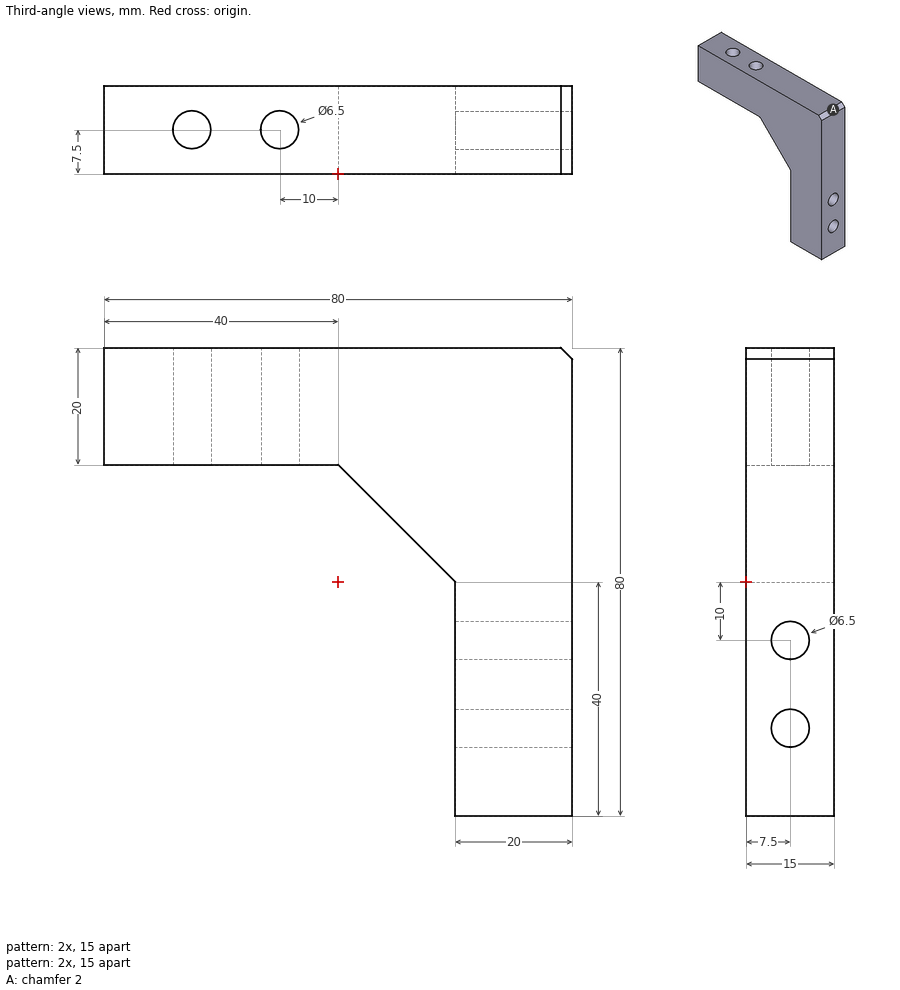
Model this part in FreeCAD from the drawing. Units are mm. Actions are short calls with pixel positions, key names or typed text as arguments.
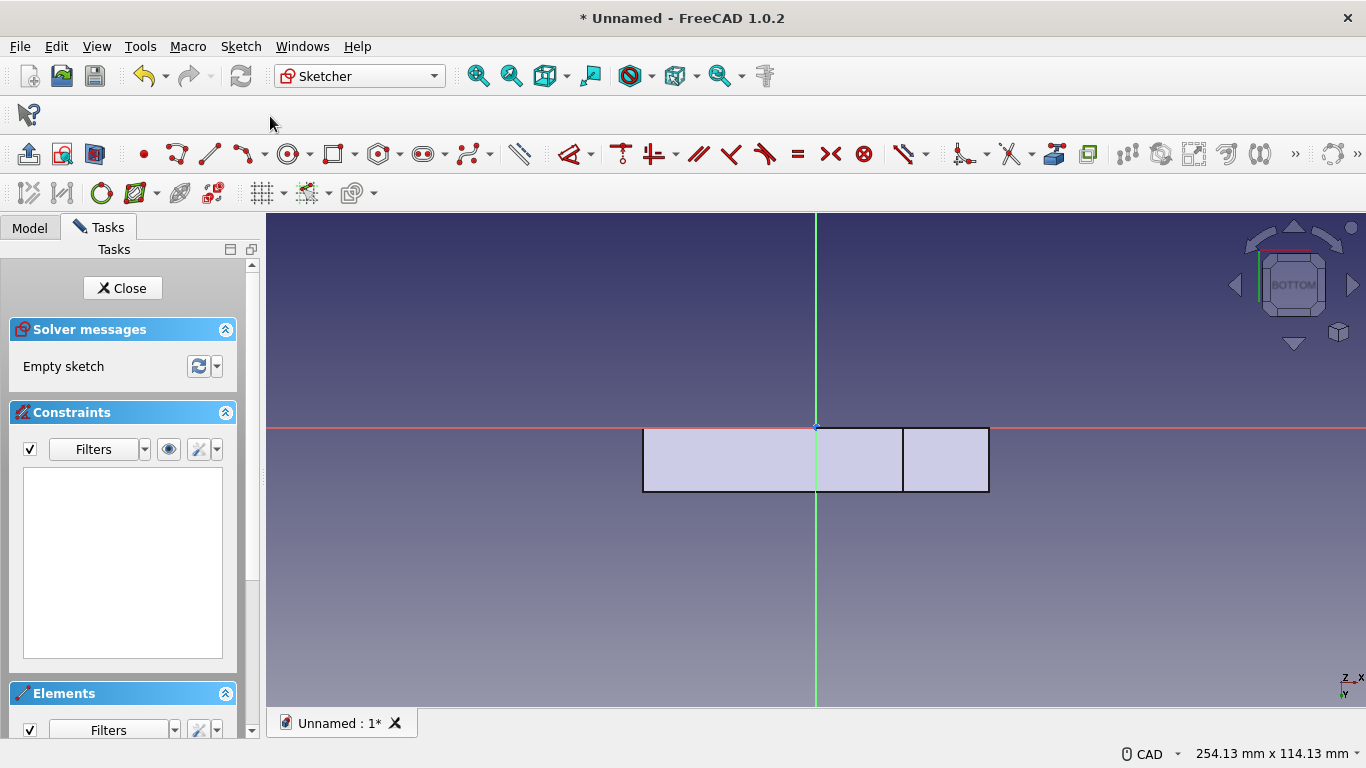
key(q)
key(s)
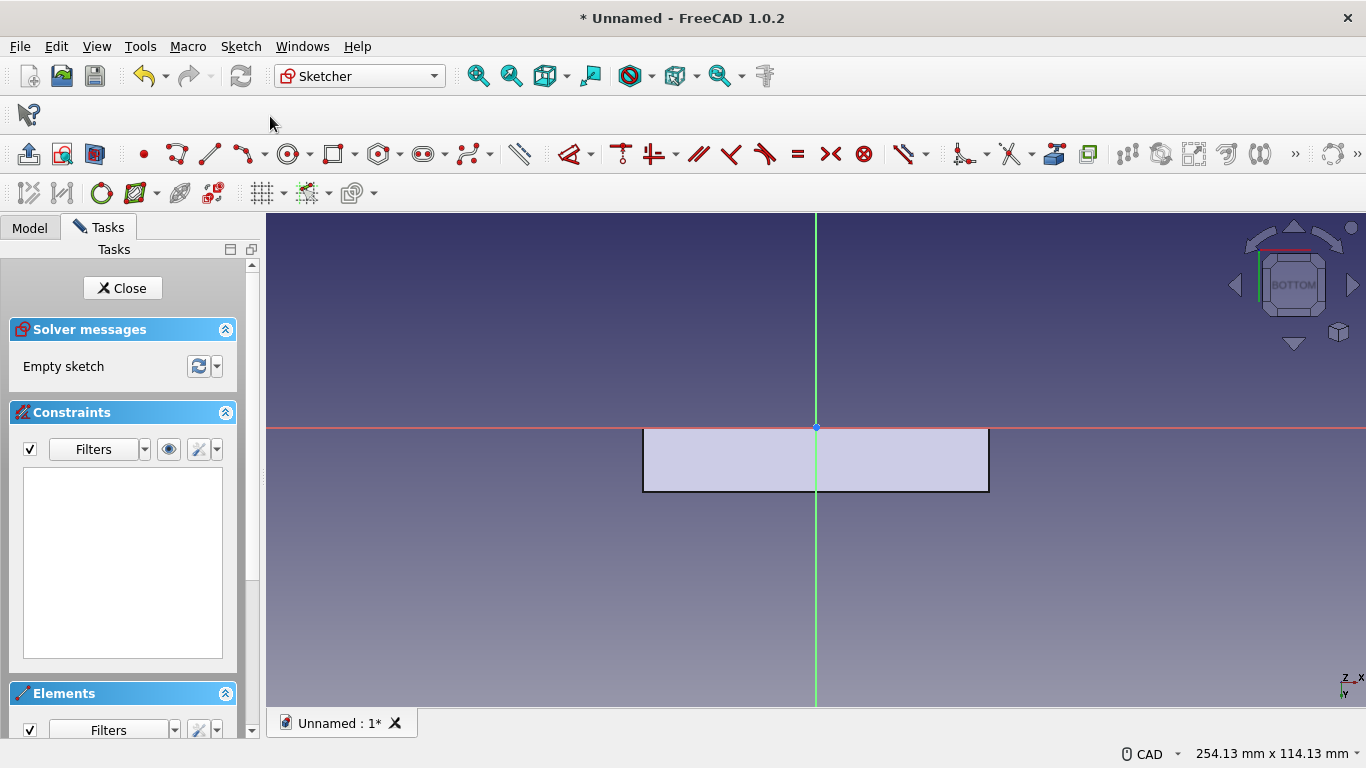
scroll(795, 449, up, 9)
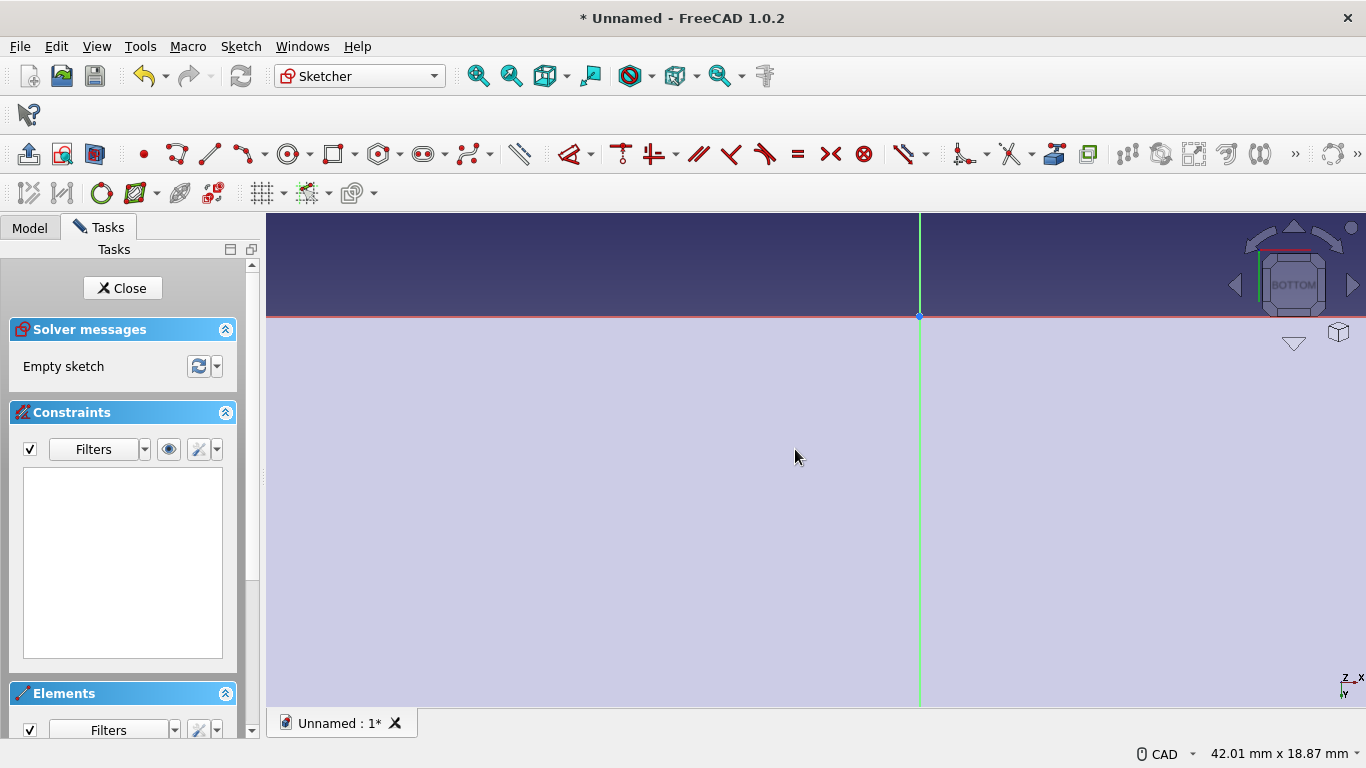
key(g)
key(c)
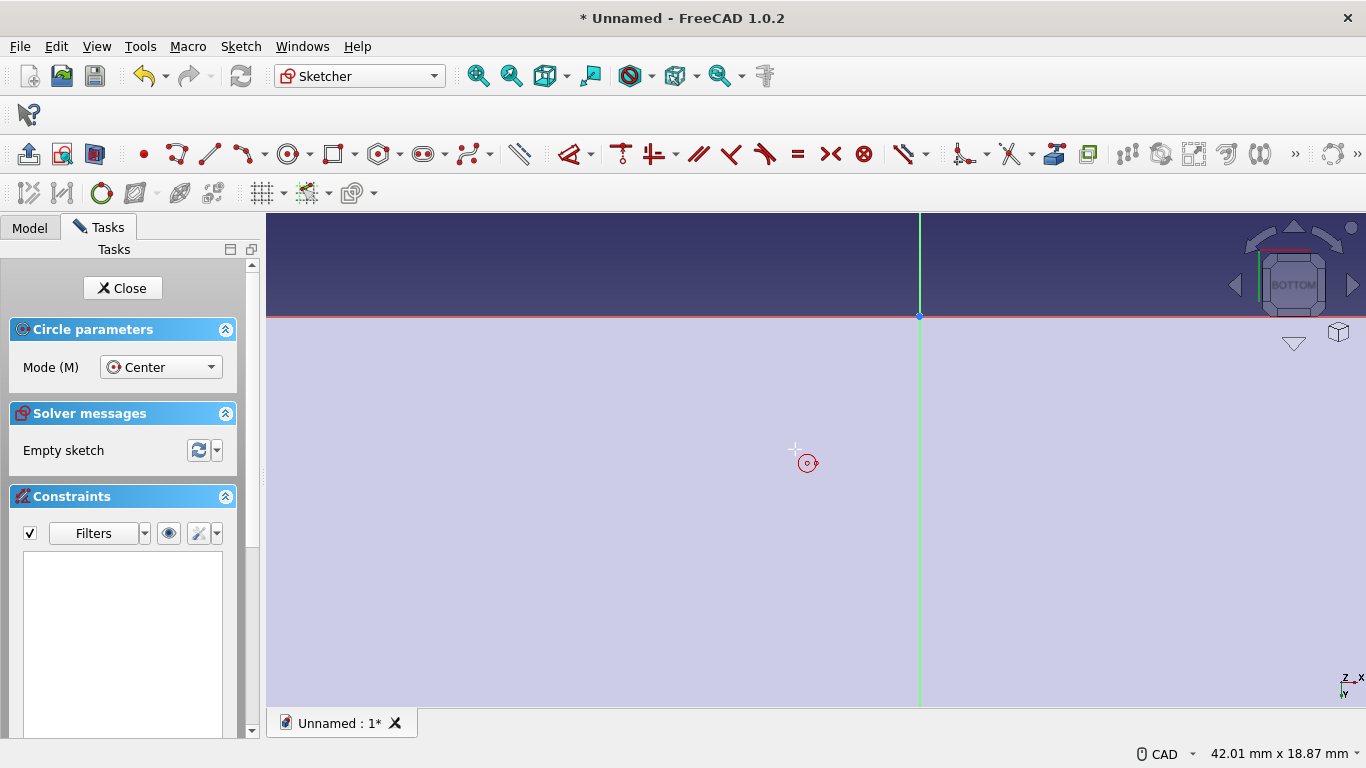
click(658, 513)
move(718, 453)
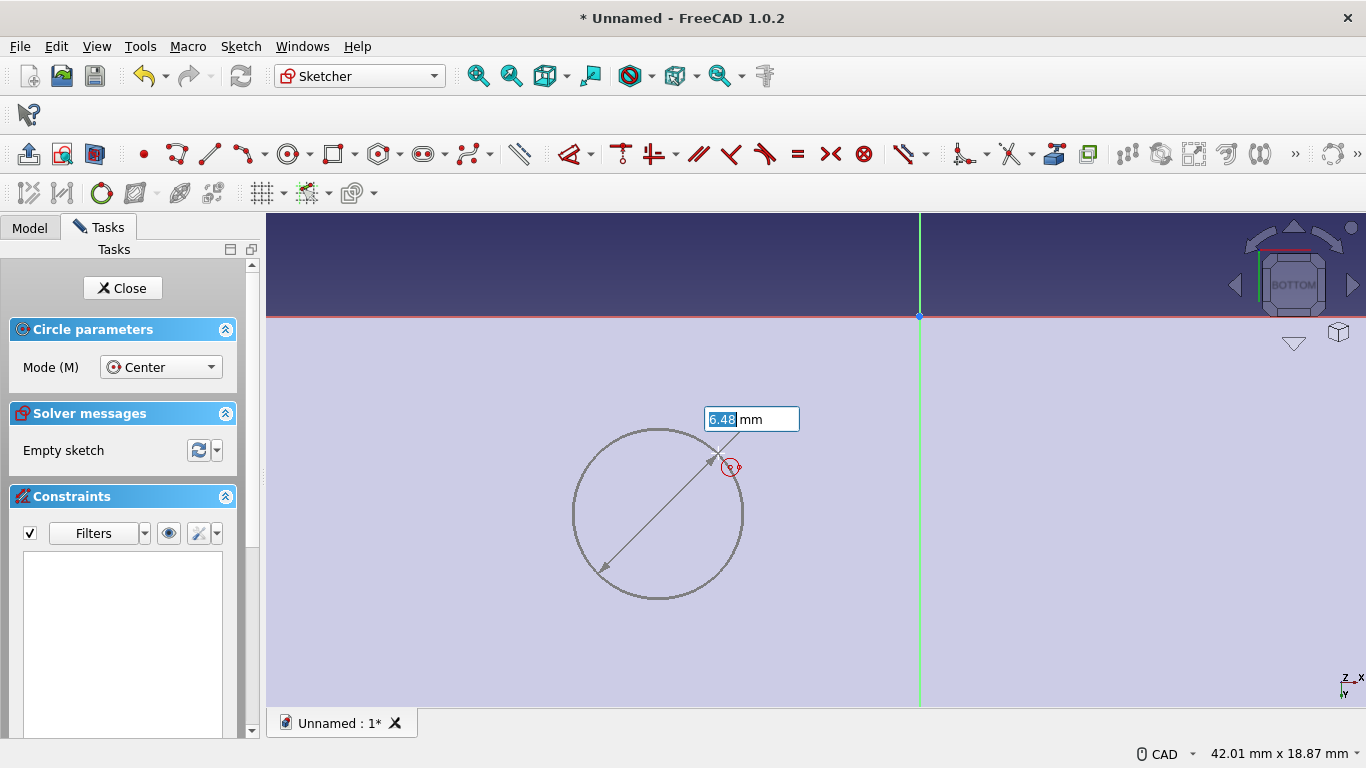
text(6.5)
key(Return)
key(Escape)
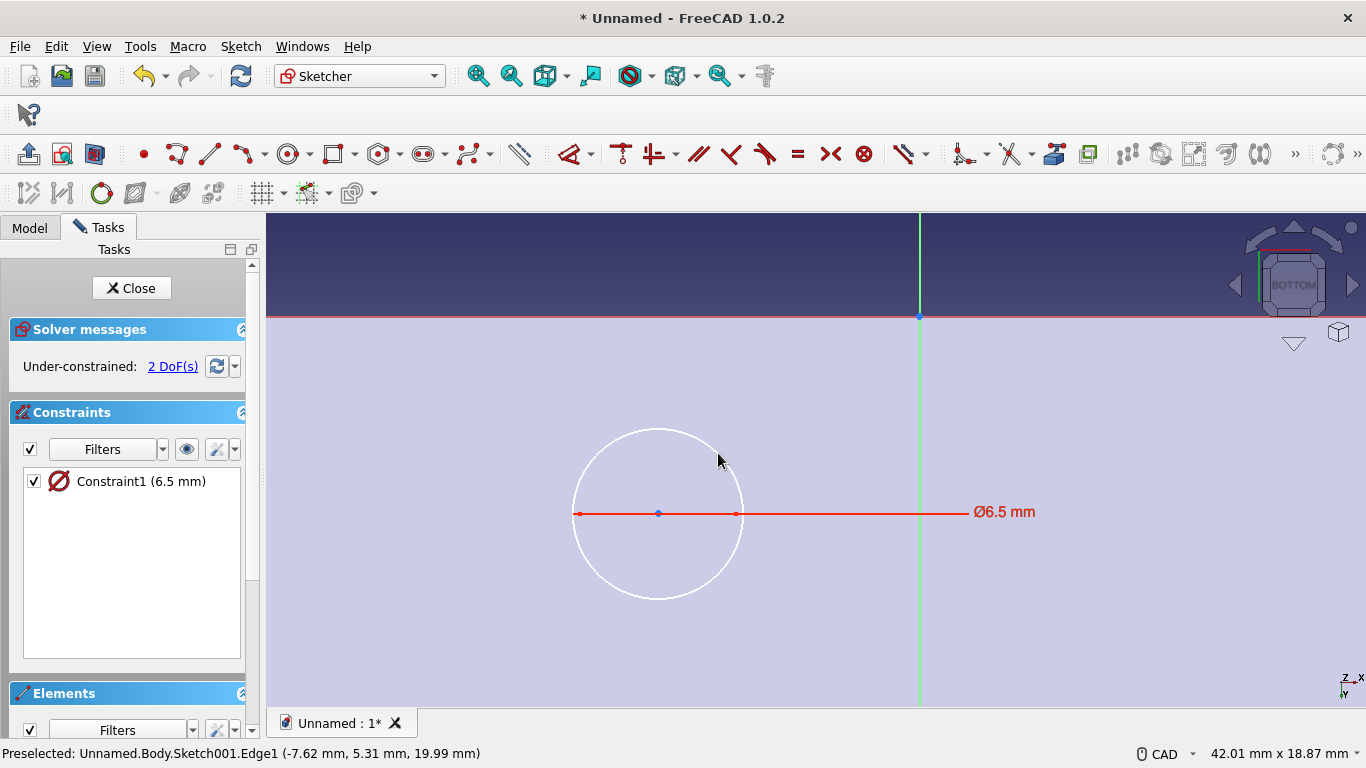
click(568, 154)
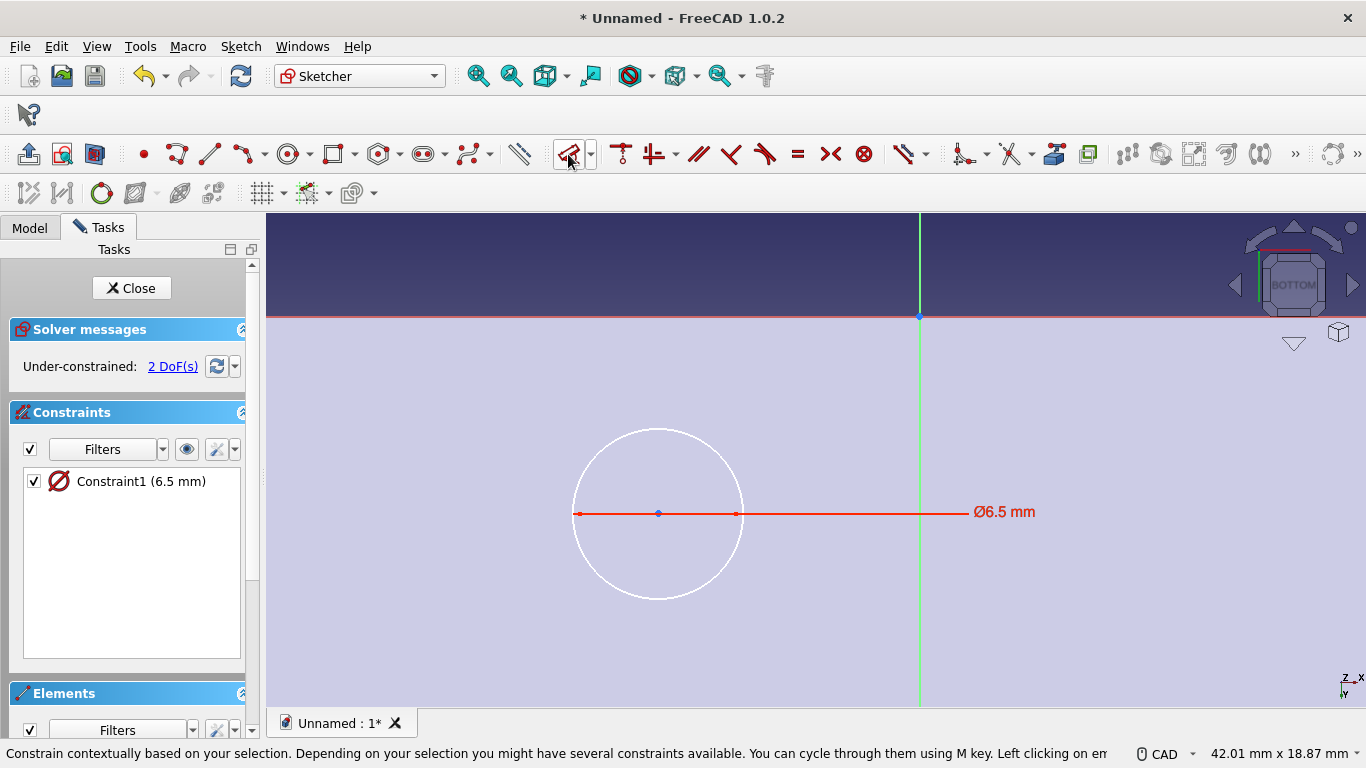
click(658, 514)
click(789, 283)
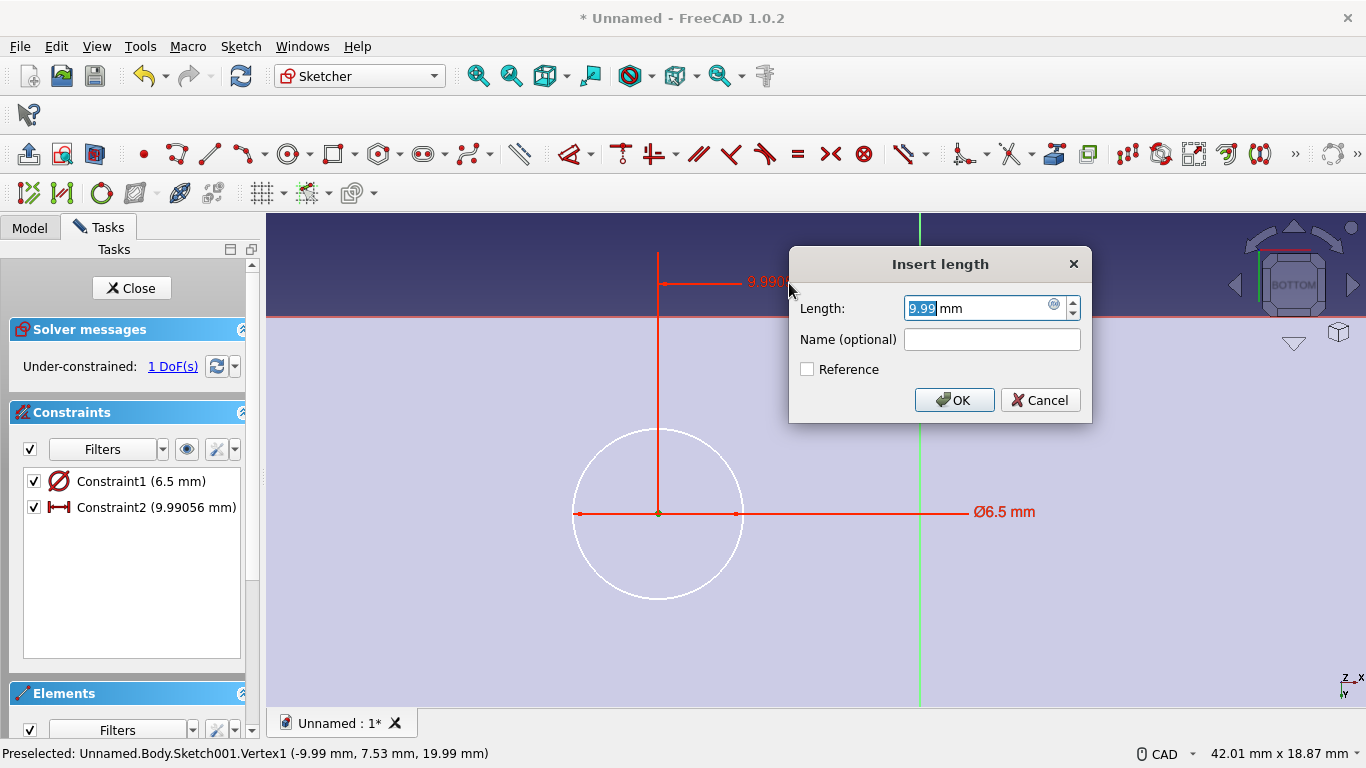
text(10)
key(Return)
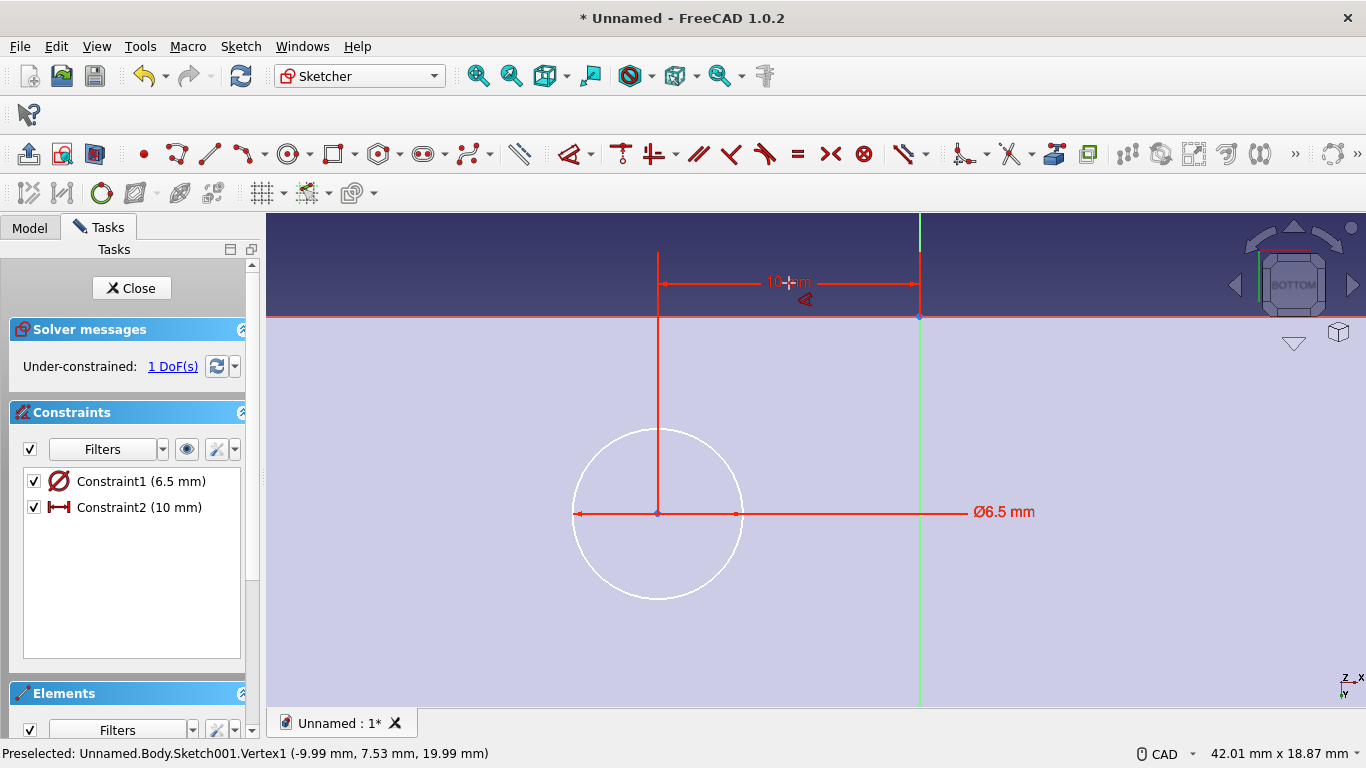
click(658, 514)
click(954, 415)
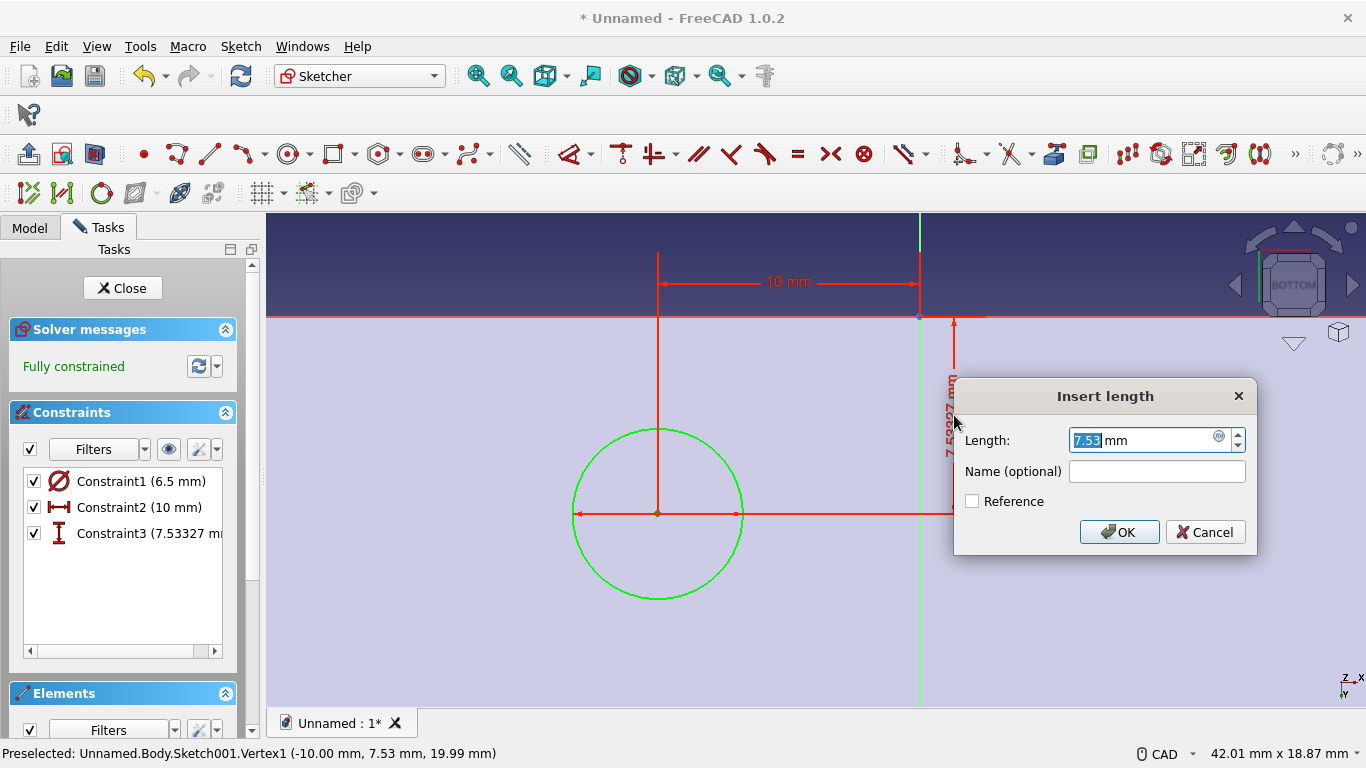
text(7.5)
key(Return)
key(Escape)